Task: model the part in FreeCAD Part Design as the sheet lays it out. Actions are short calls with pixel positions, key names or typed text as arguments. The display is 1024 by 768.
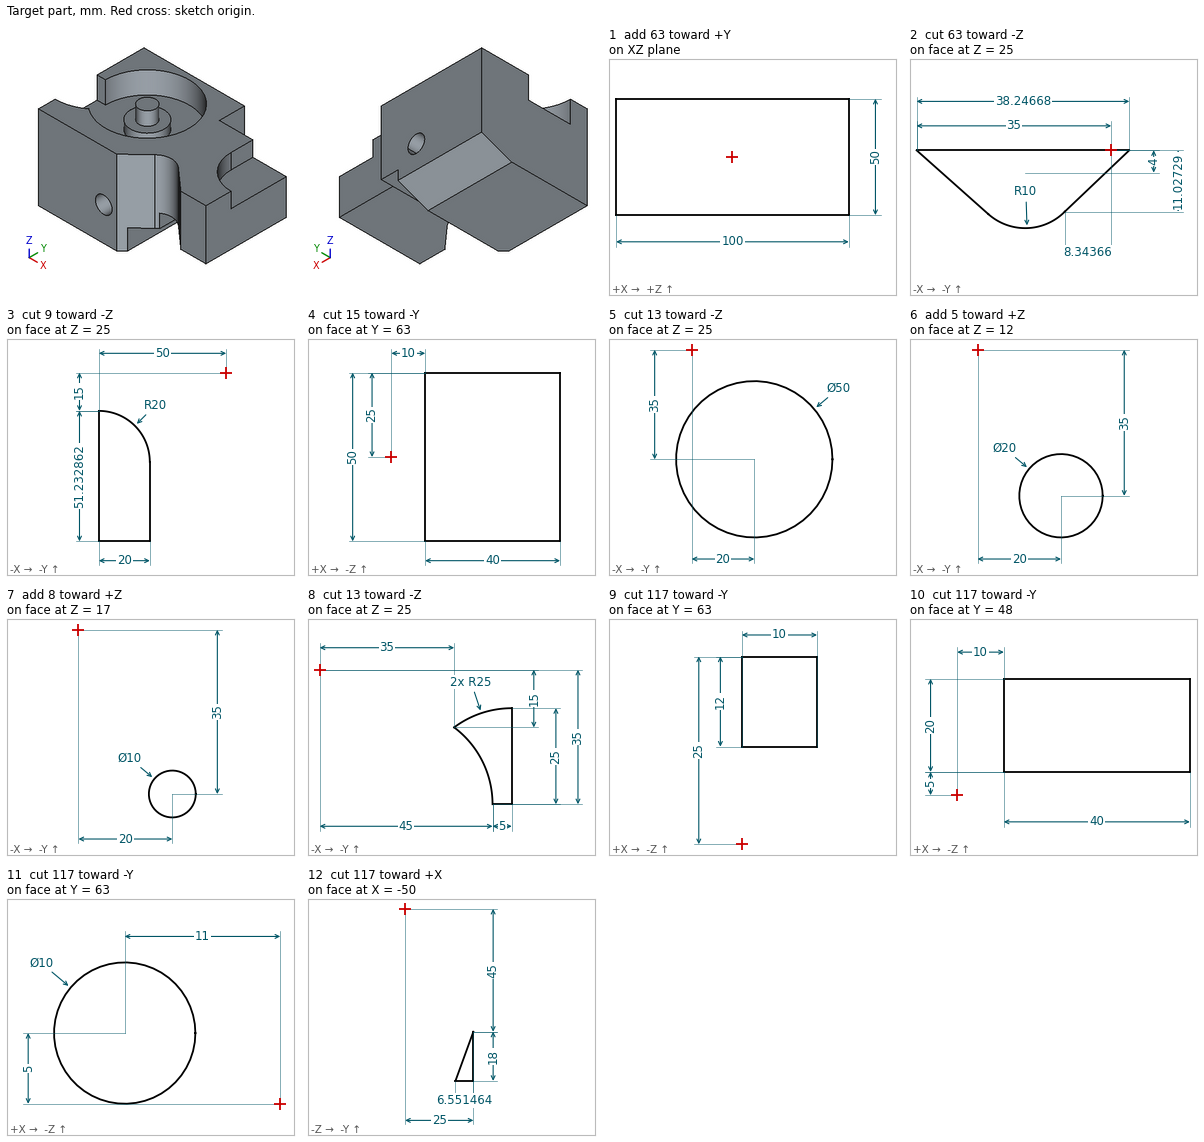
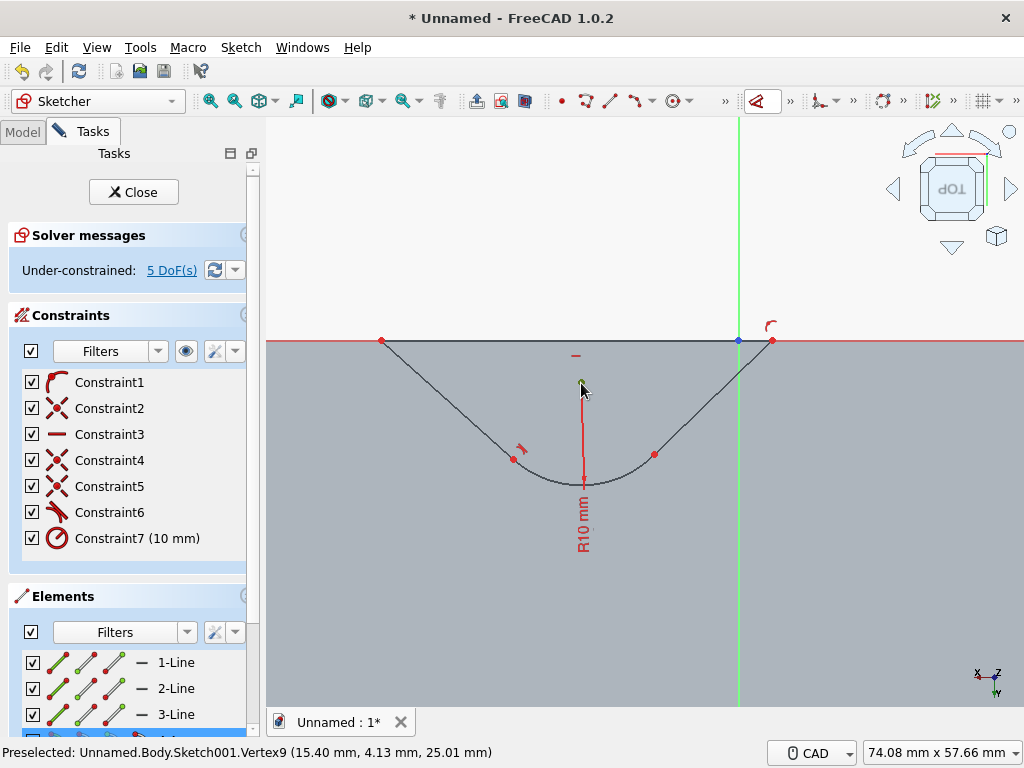
click(776, 102)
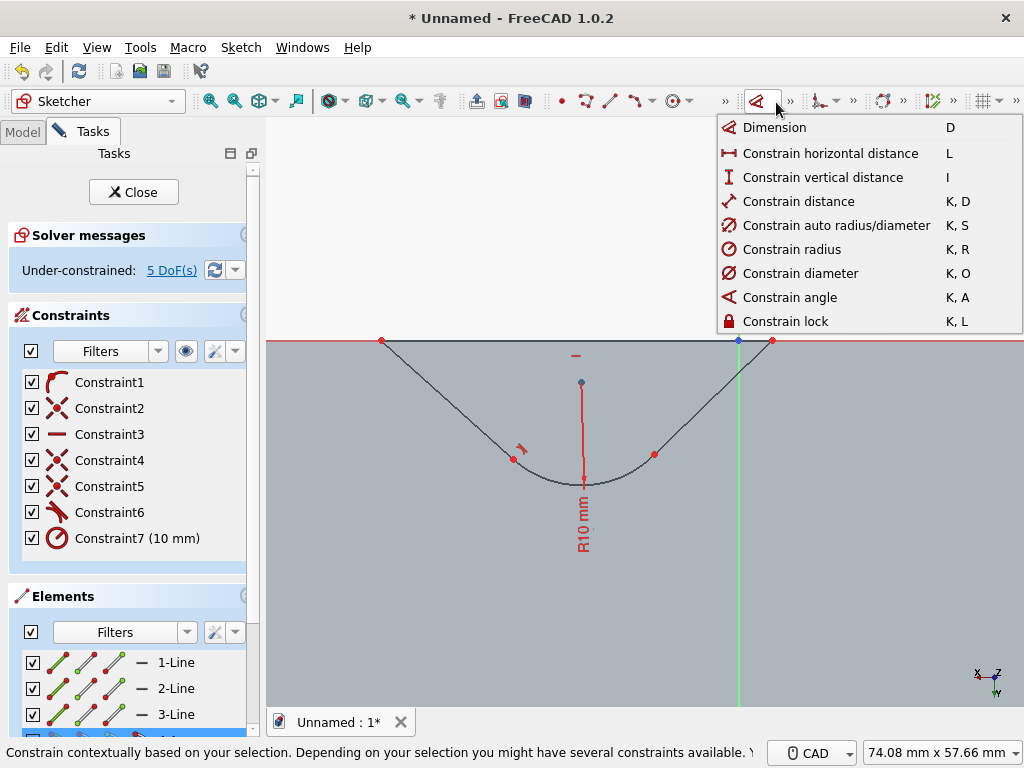
click(870, 177)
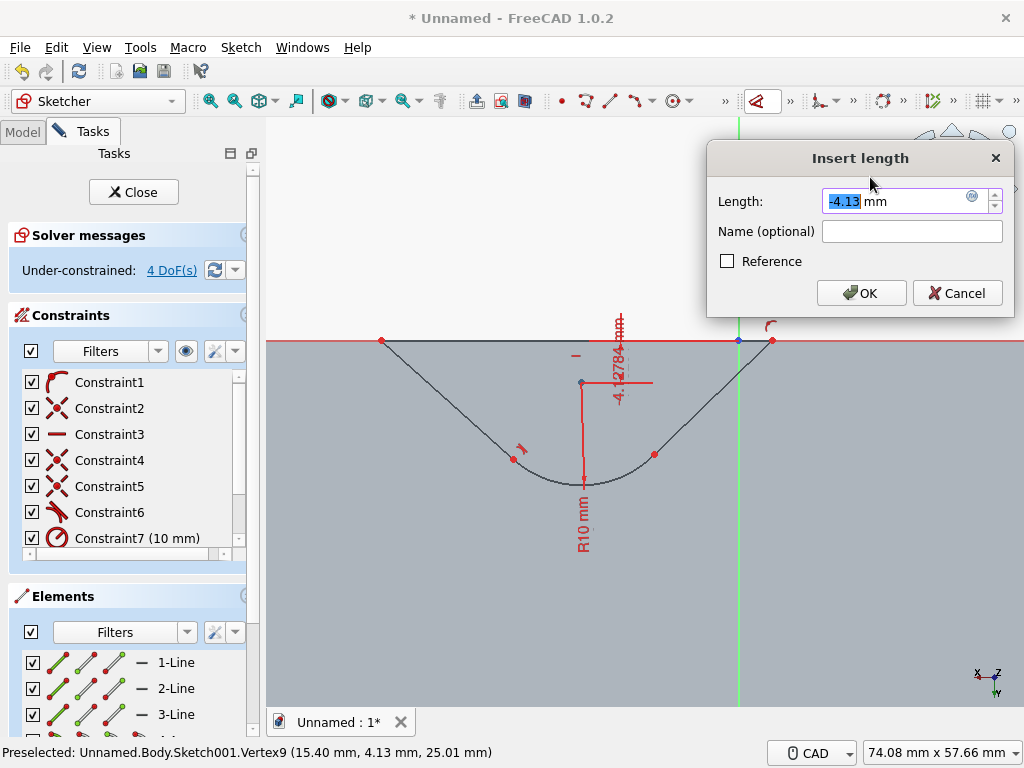
text(-4)
key(Return)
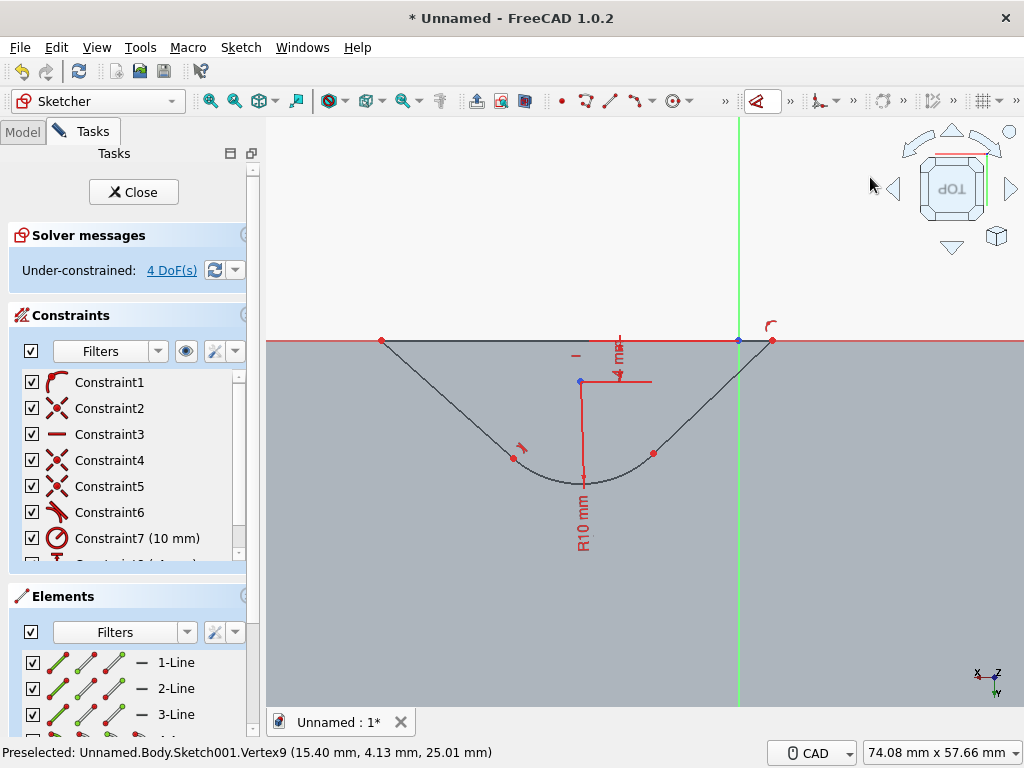
click(381, 341)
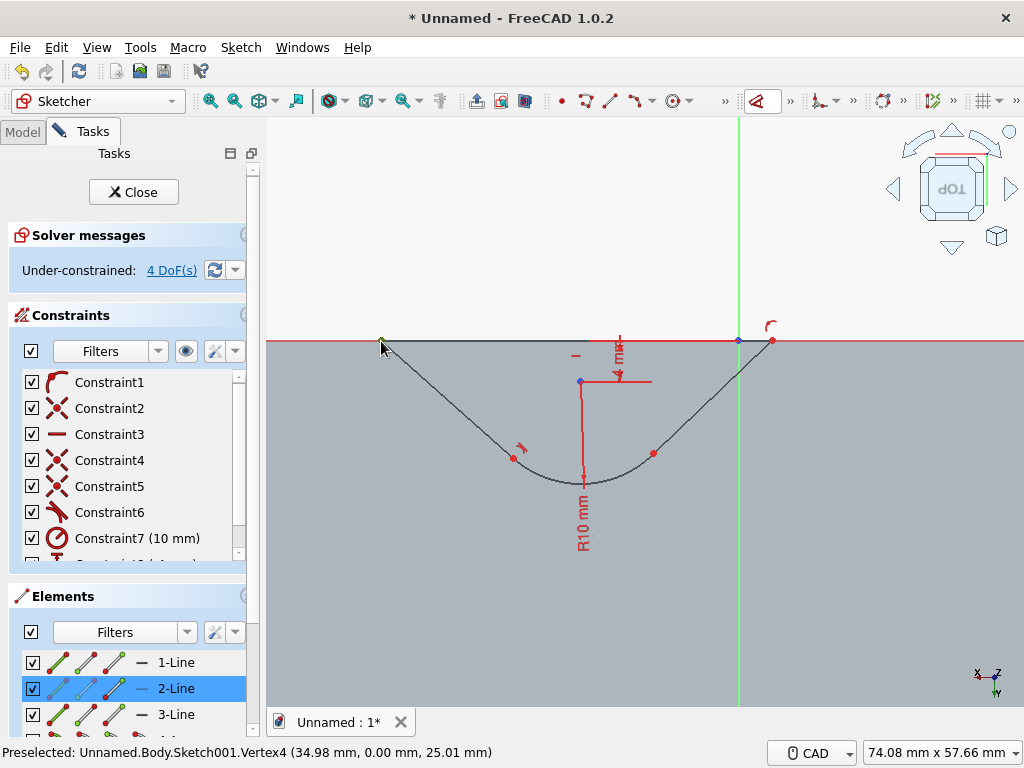
click(776, 102)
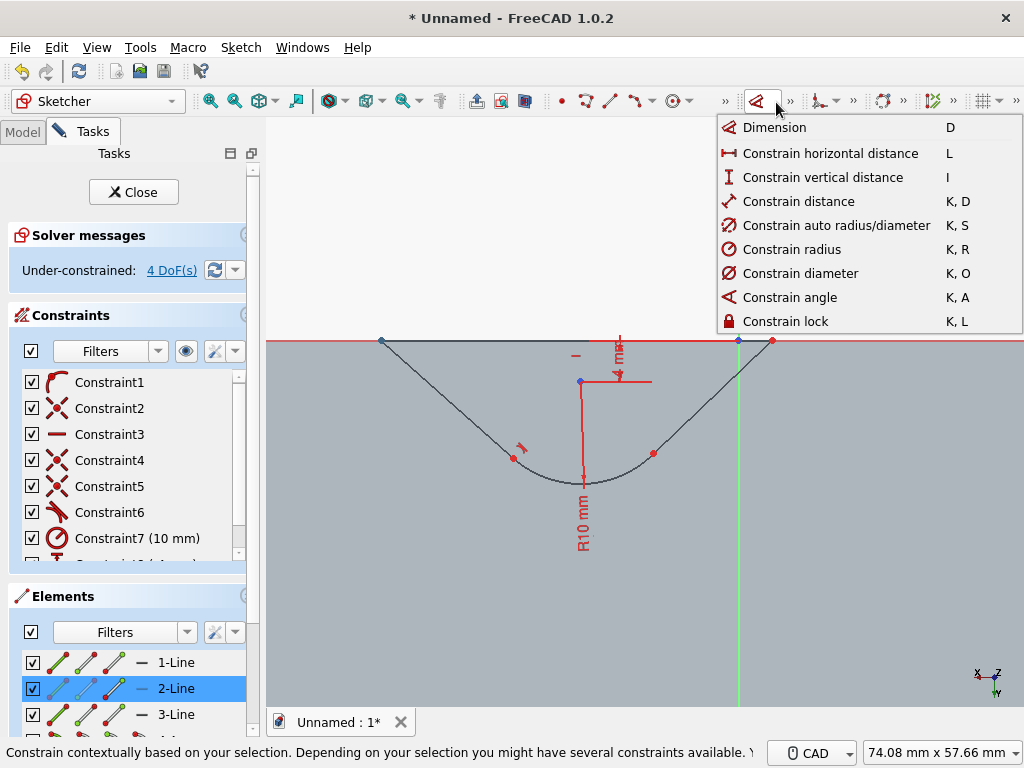
click(870, 153)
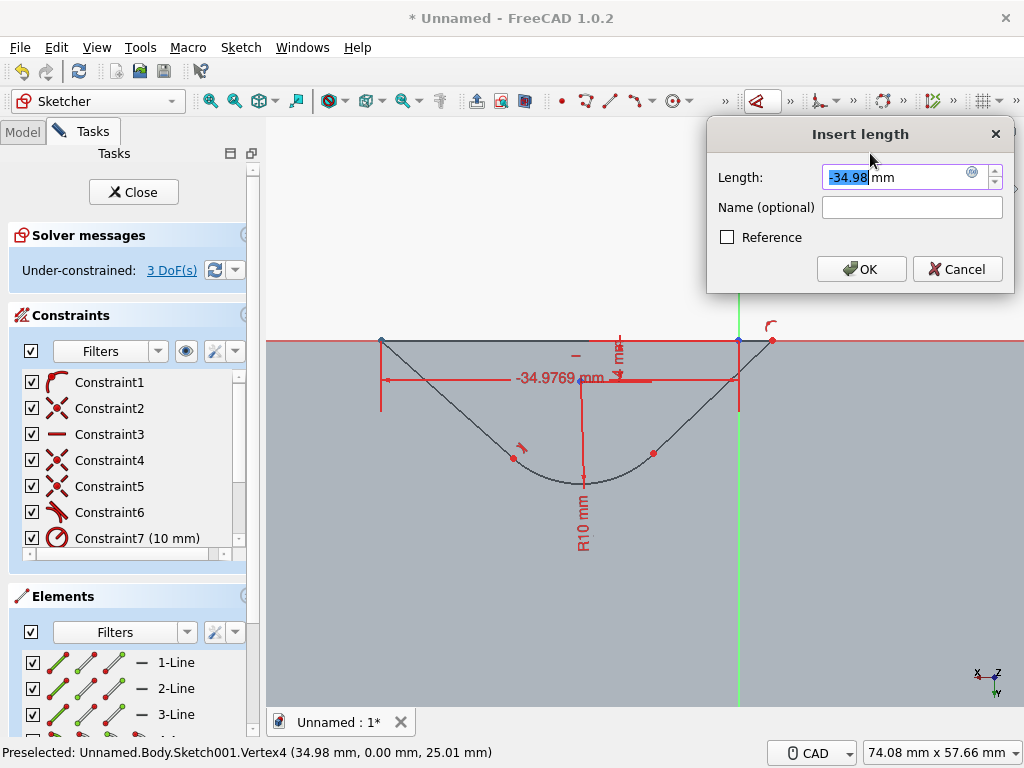
text(-35)
key(Return)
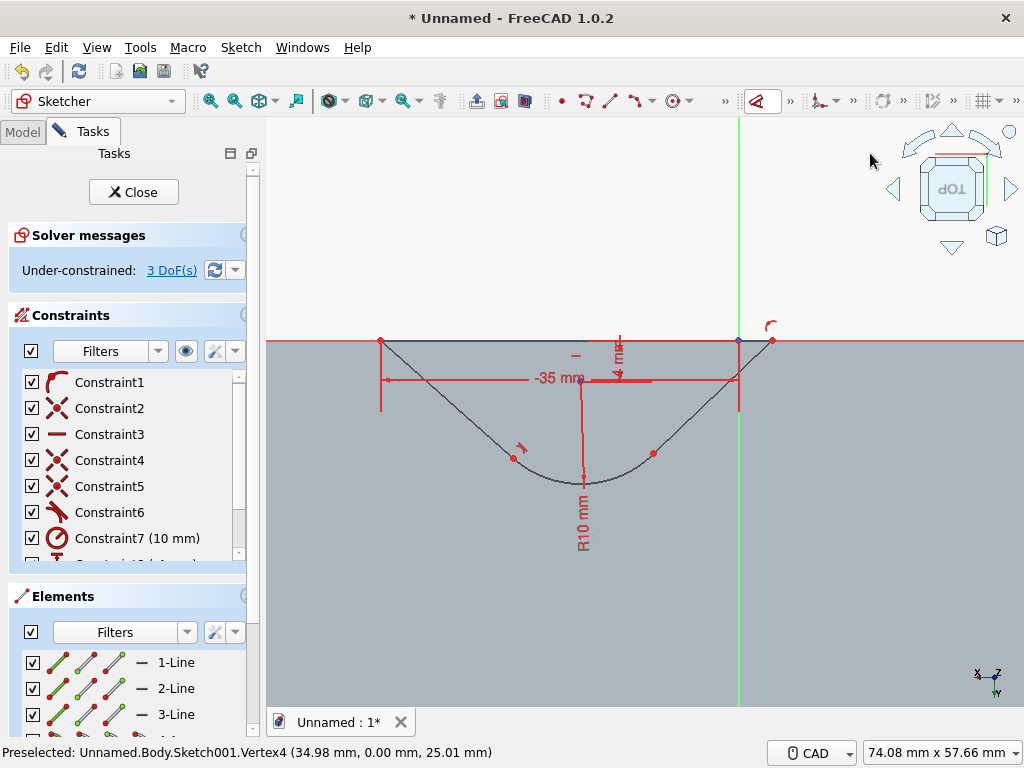
click(655, 341)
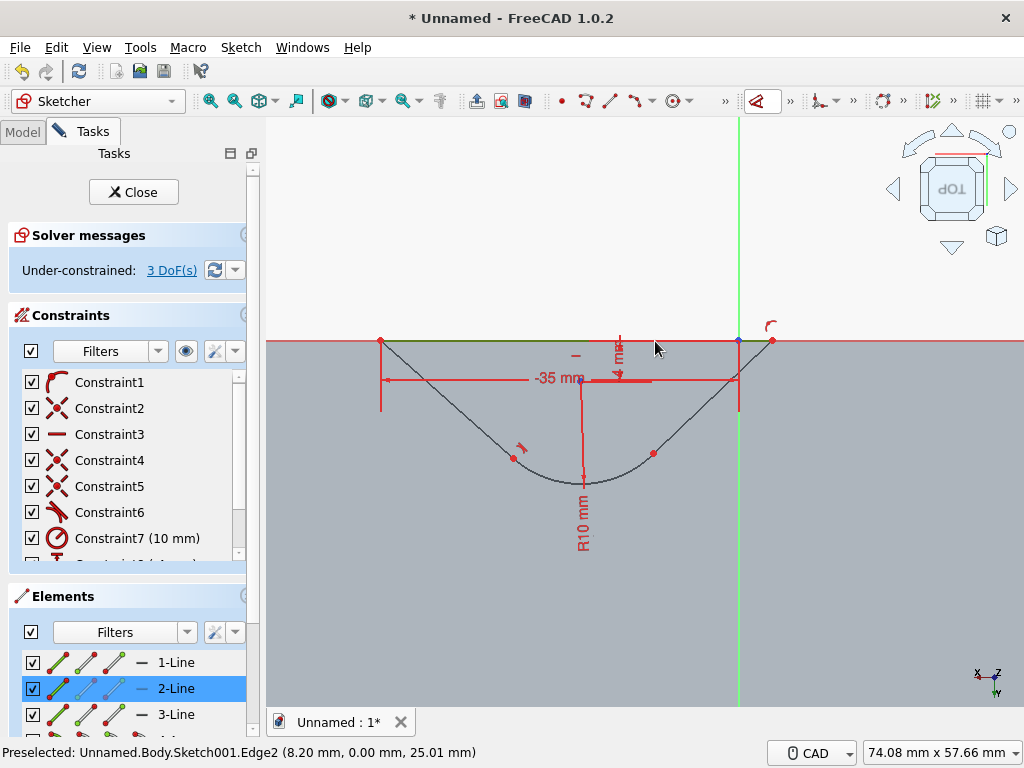
click(776, 102)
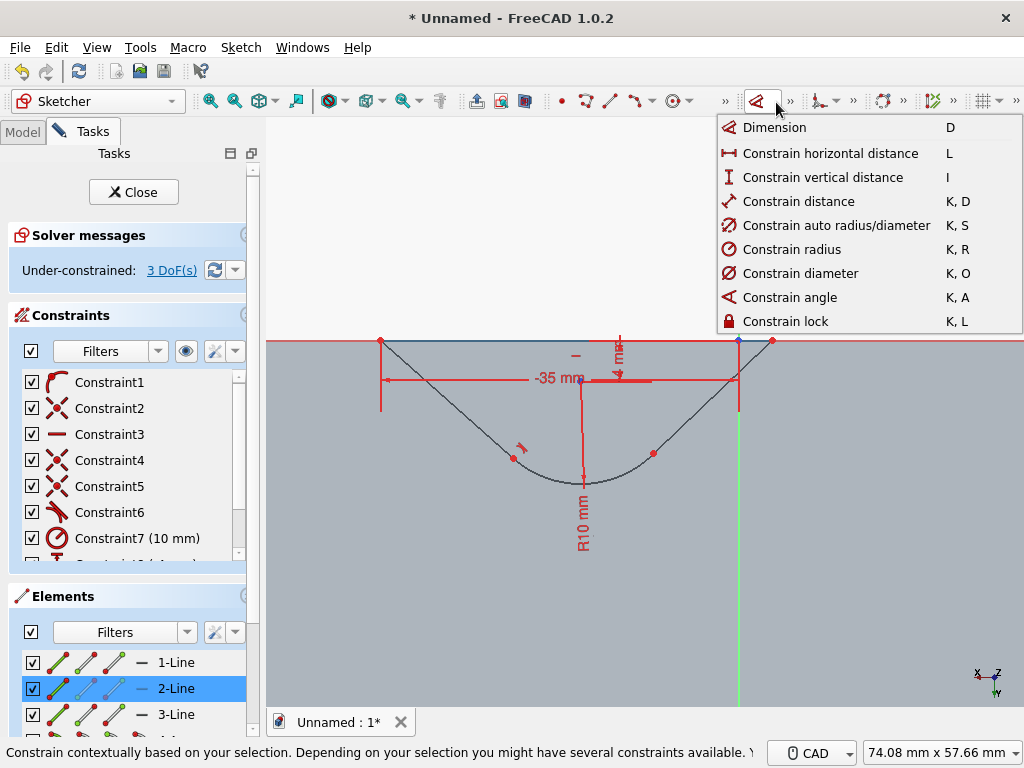
click(870, 153)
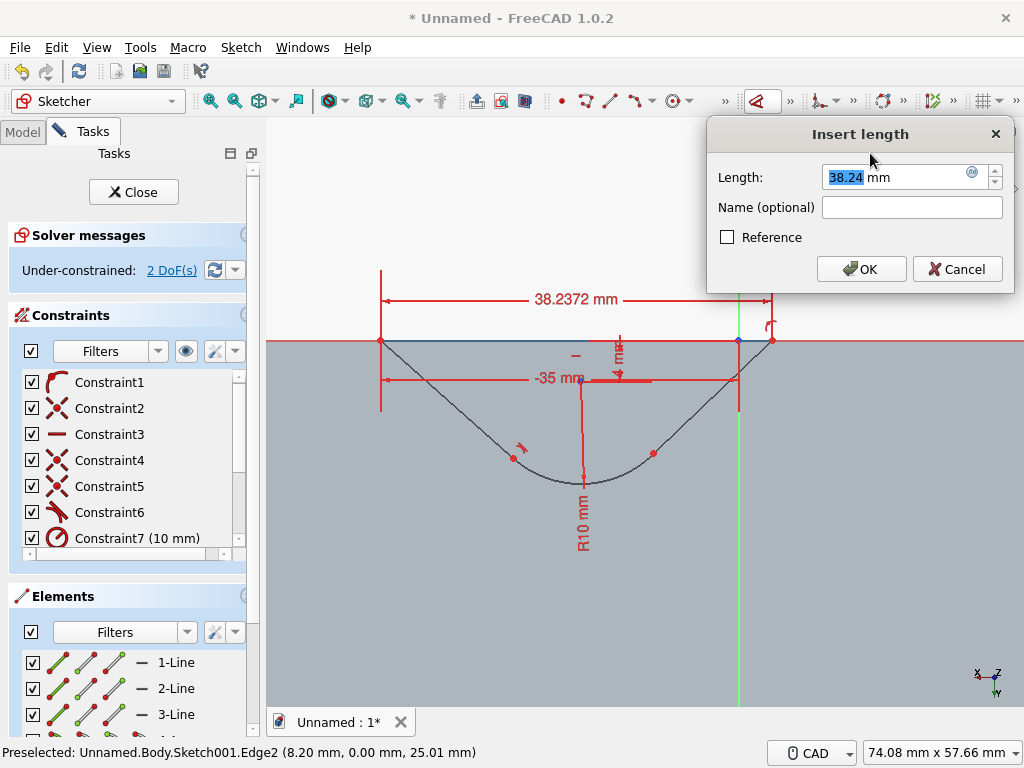
text(38.24668)
key(Return)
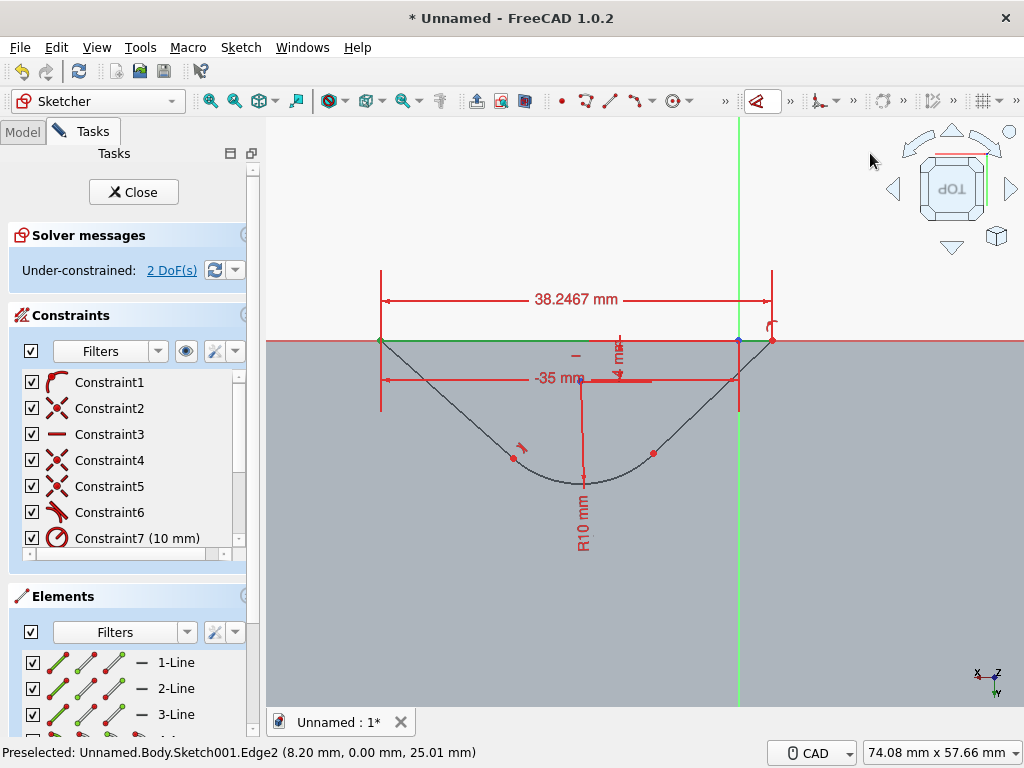
click(653, 454)